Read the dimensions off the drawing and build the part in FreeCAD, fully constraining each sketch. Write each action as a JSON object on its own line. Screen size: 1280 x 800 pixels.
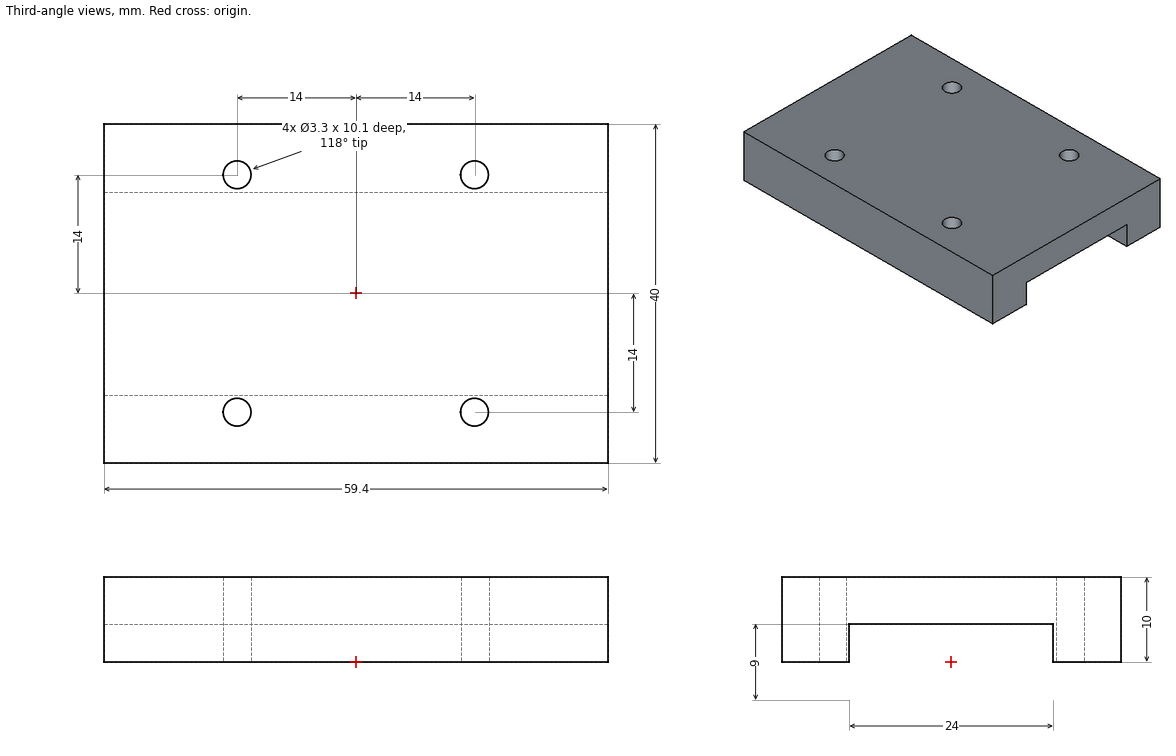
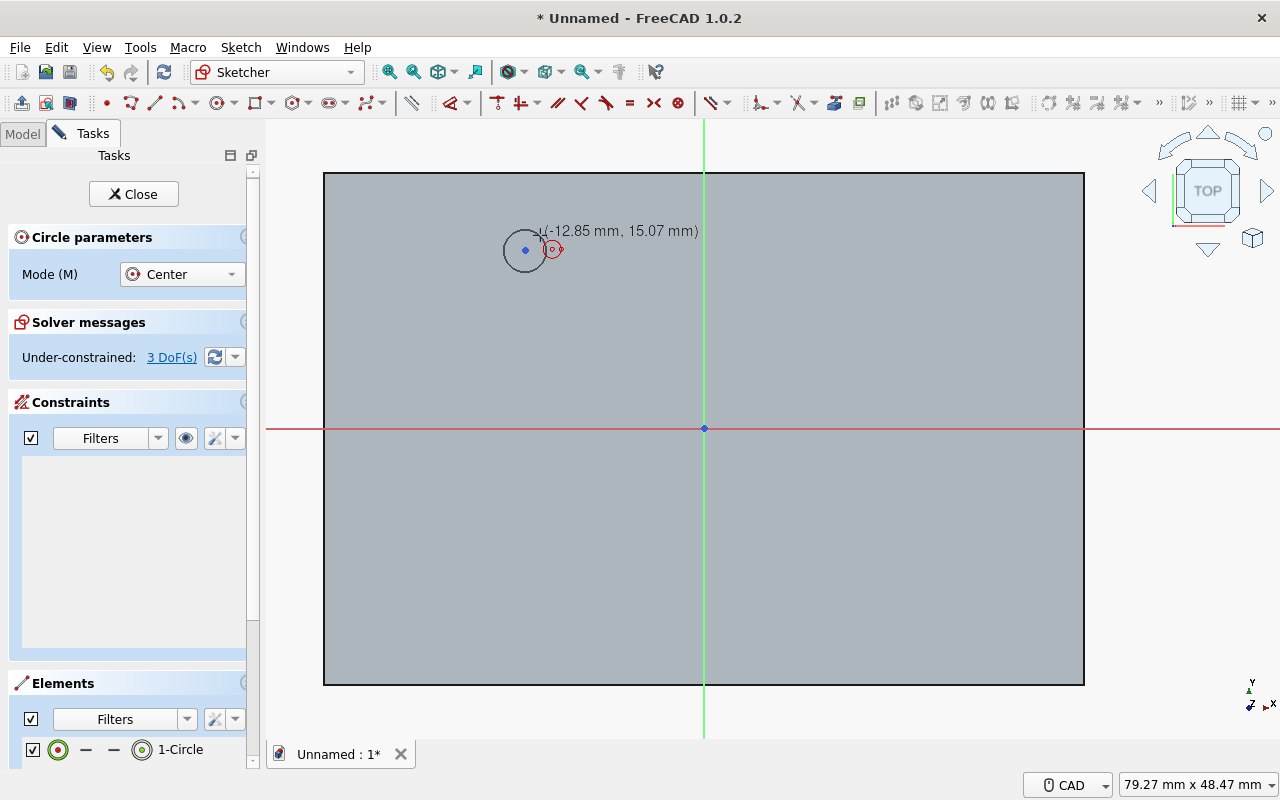
{"action": "left_click", "coordinate": [883, 250]}
{"action": "left_click", "coordinate": [898, 235]}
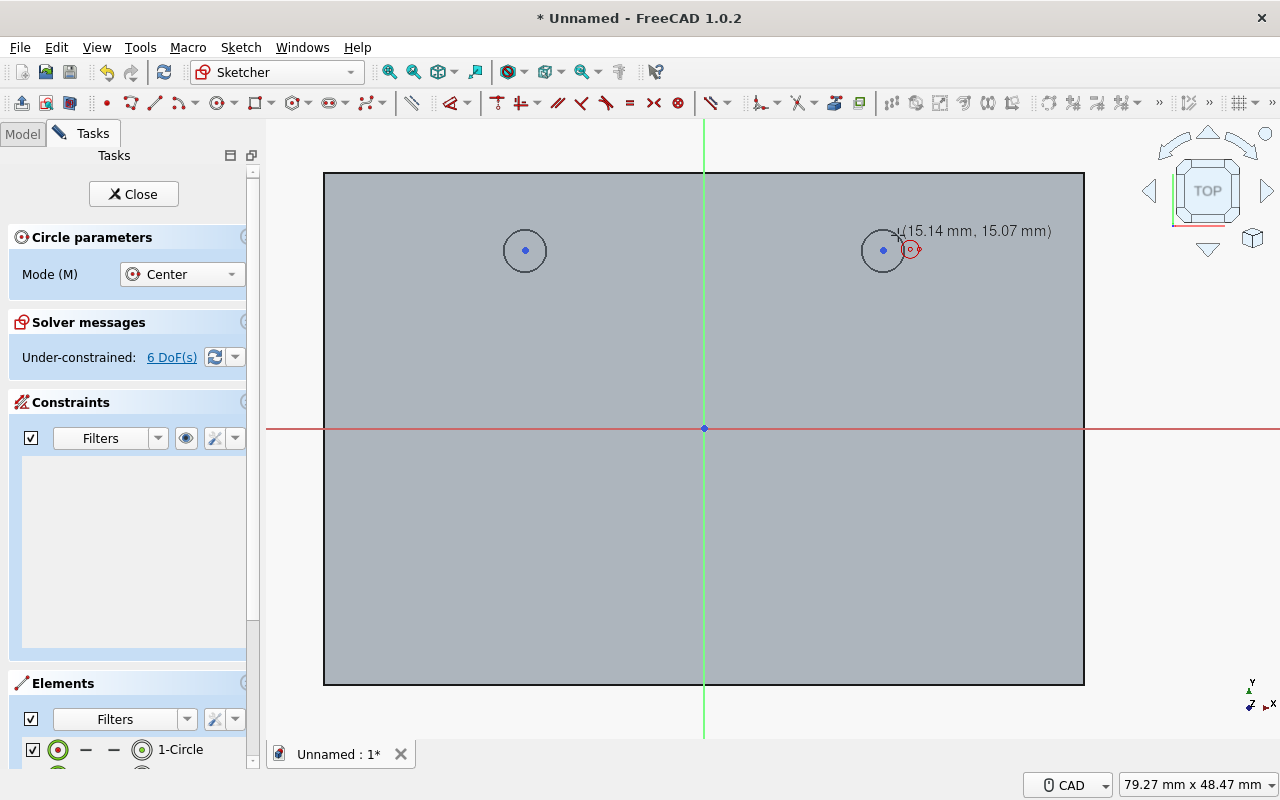
{"action": "left_click", "coordinate": [883, 608]}
{"action": "left_click", "coordinate": [898, 593]}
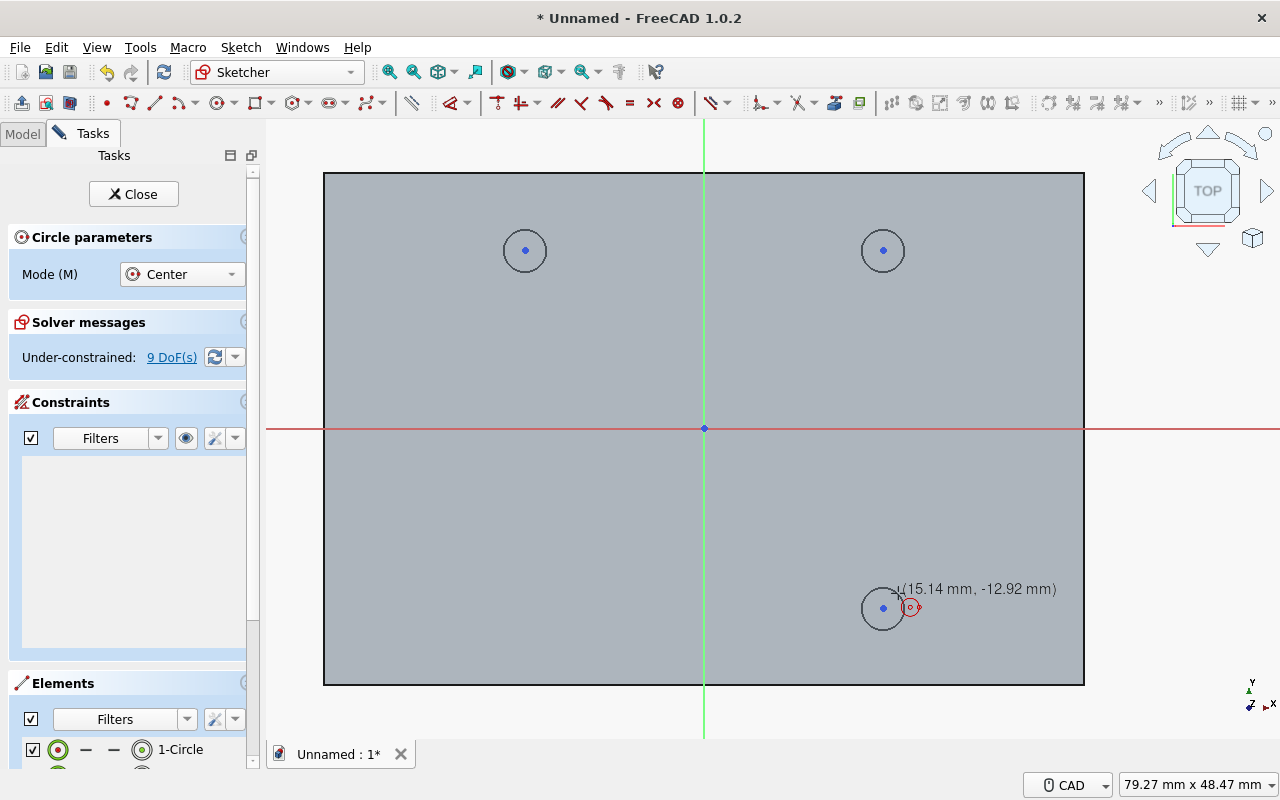
{"action": "left_click", "coordinate": [525, 608]}
{"action": "left_click", "coordinate": [540, 593]}
{"action": "key", "text": "Escape"}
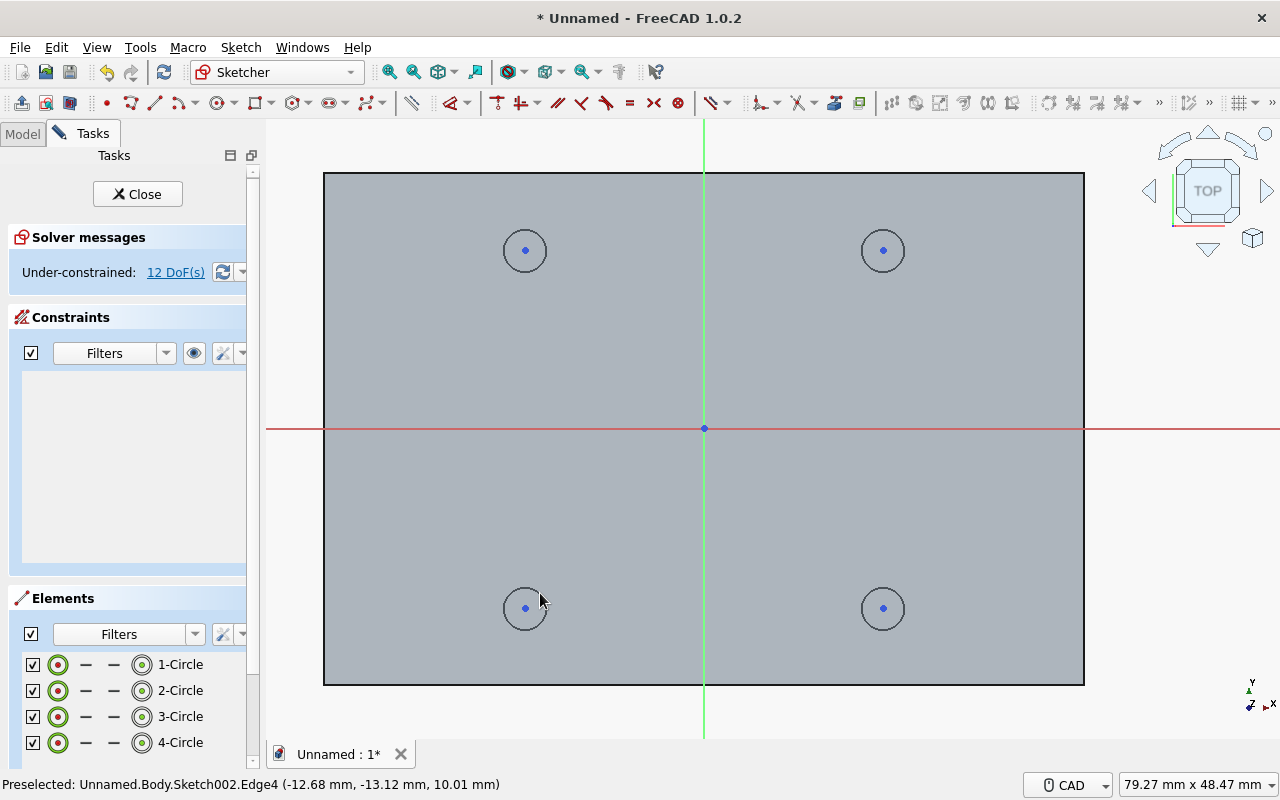
{"action": "left_click", "coordinate": [540, 236]}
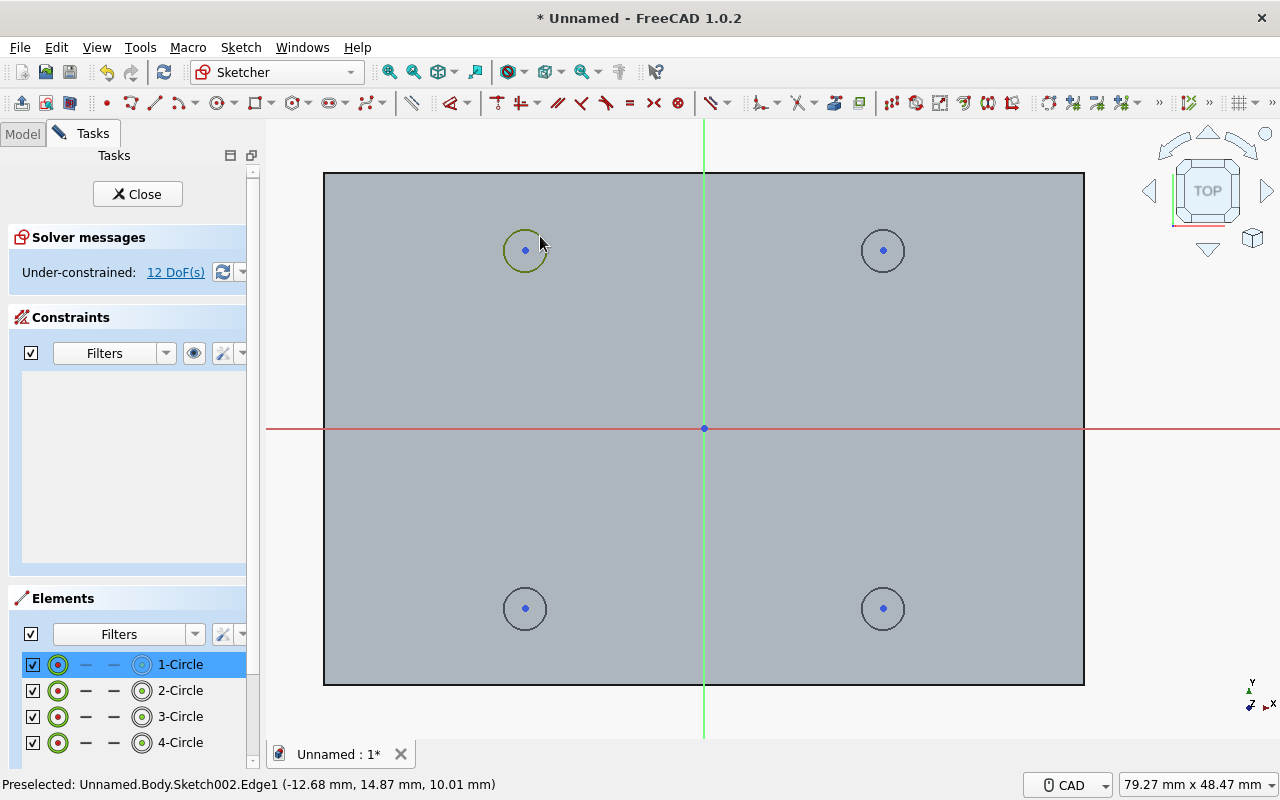
{"action": "left_click", "coordinate": [898, 236]}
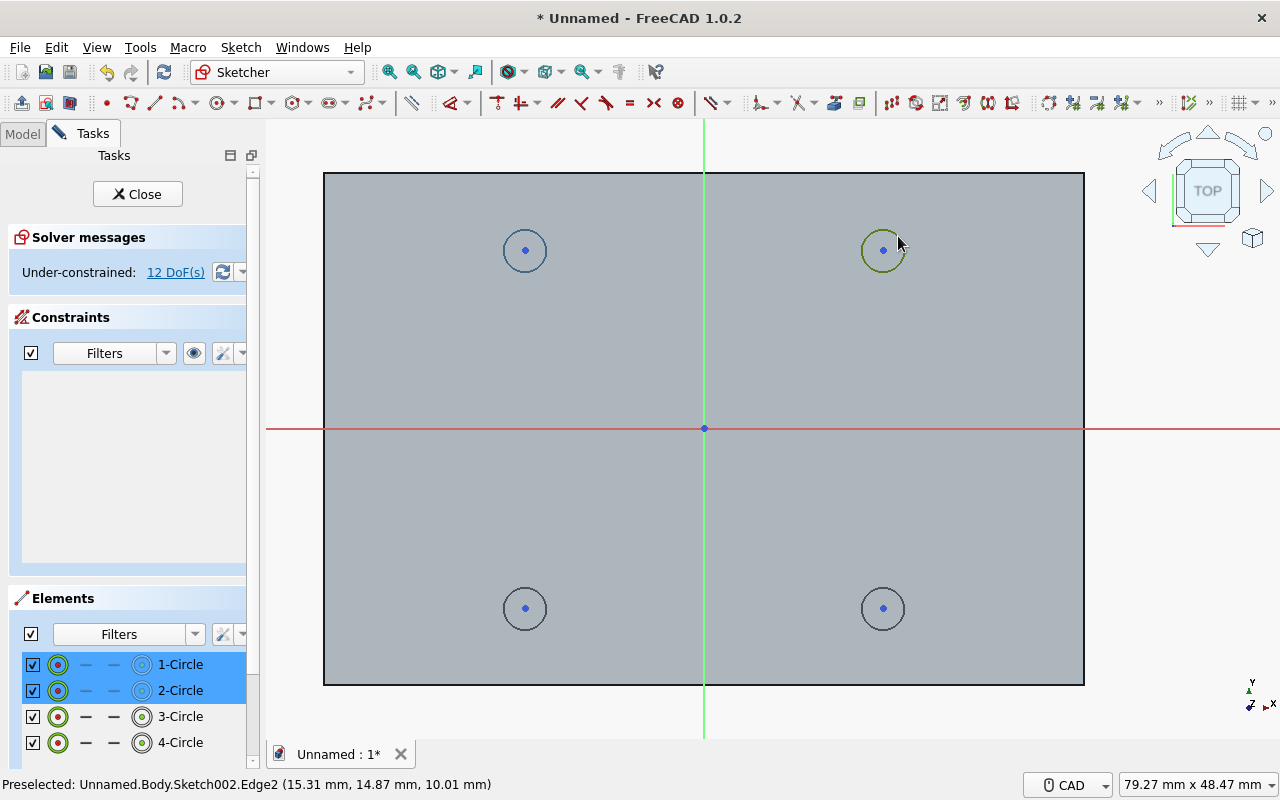
{"action": "left_click", "coordinate": [898, 594]}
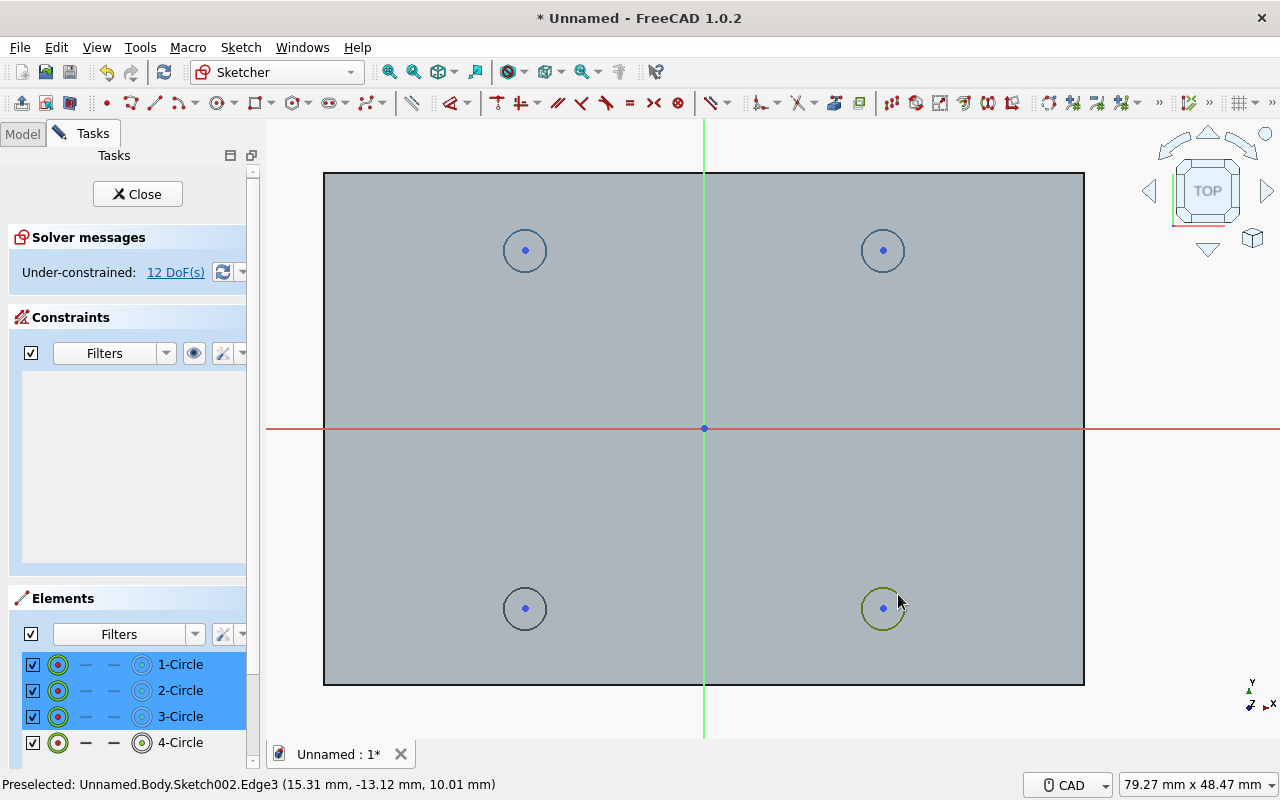
{"action": "left_click", "coordinate": [540, 594]}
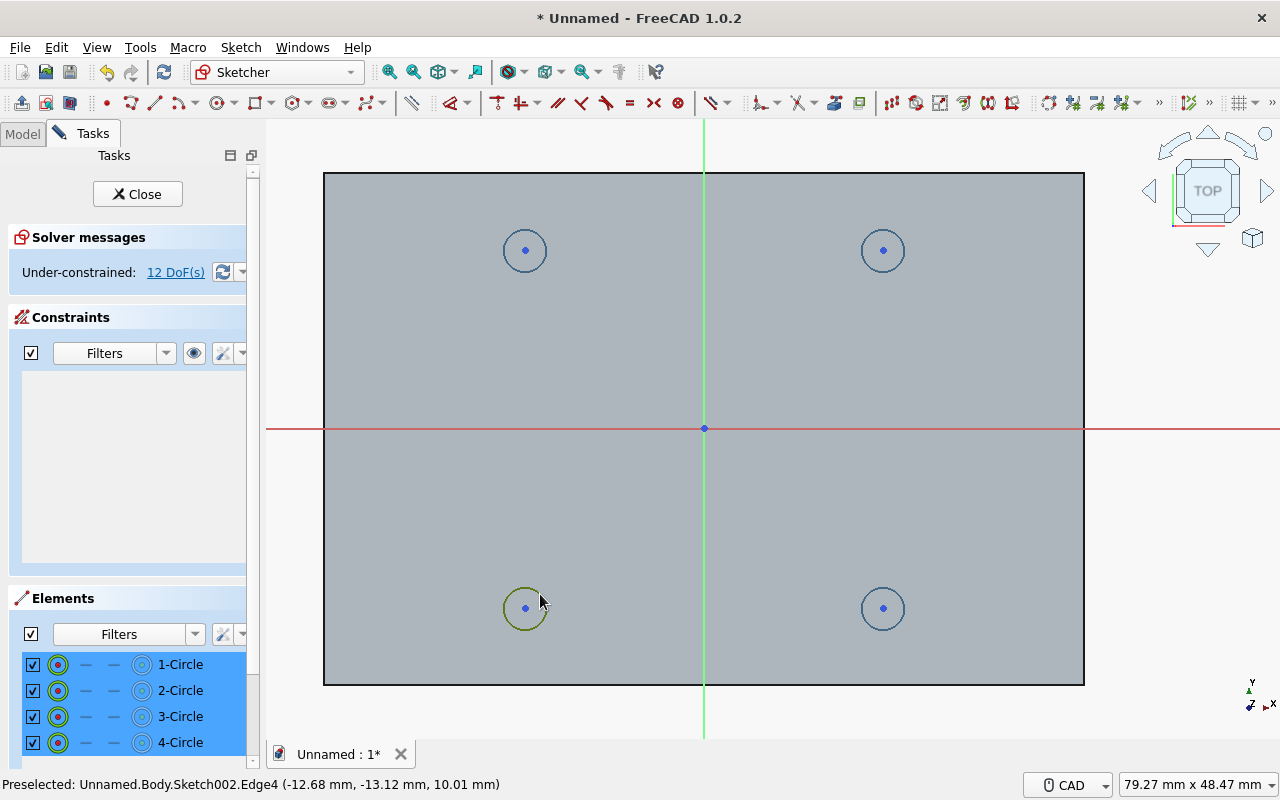
{"action": "key", "text": "e"}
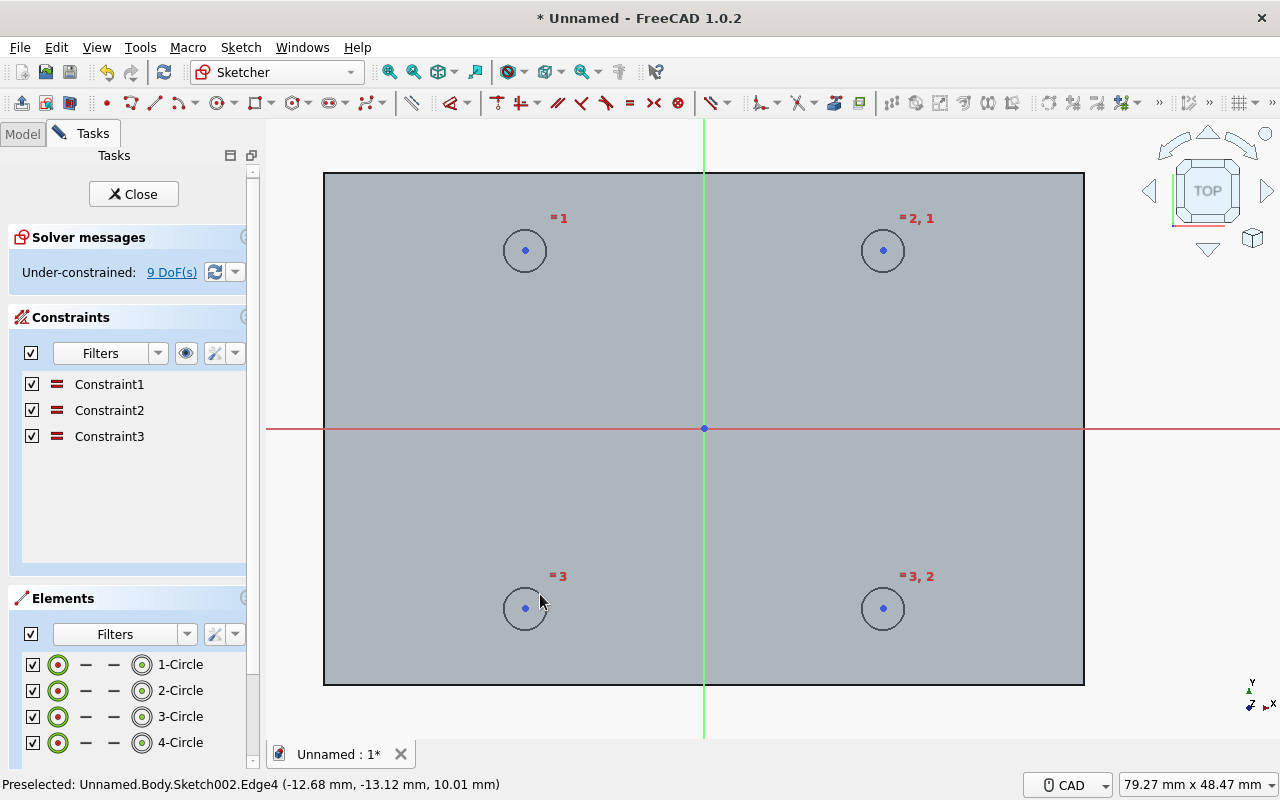
{"action": "left_click", "coordinate": [525, 251]}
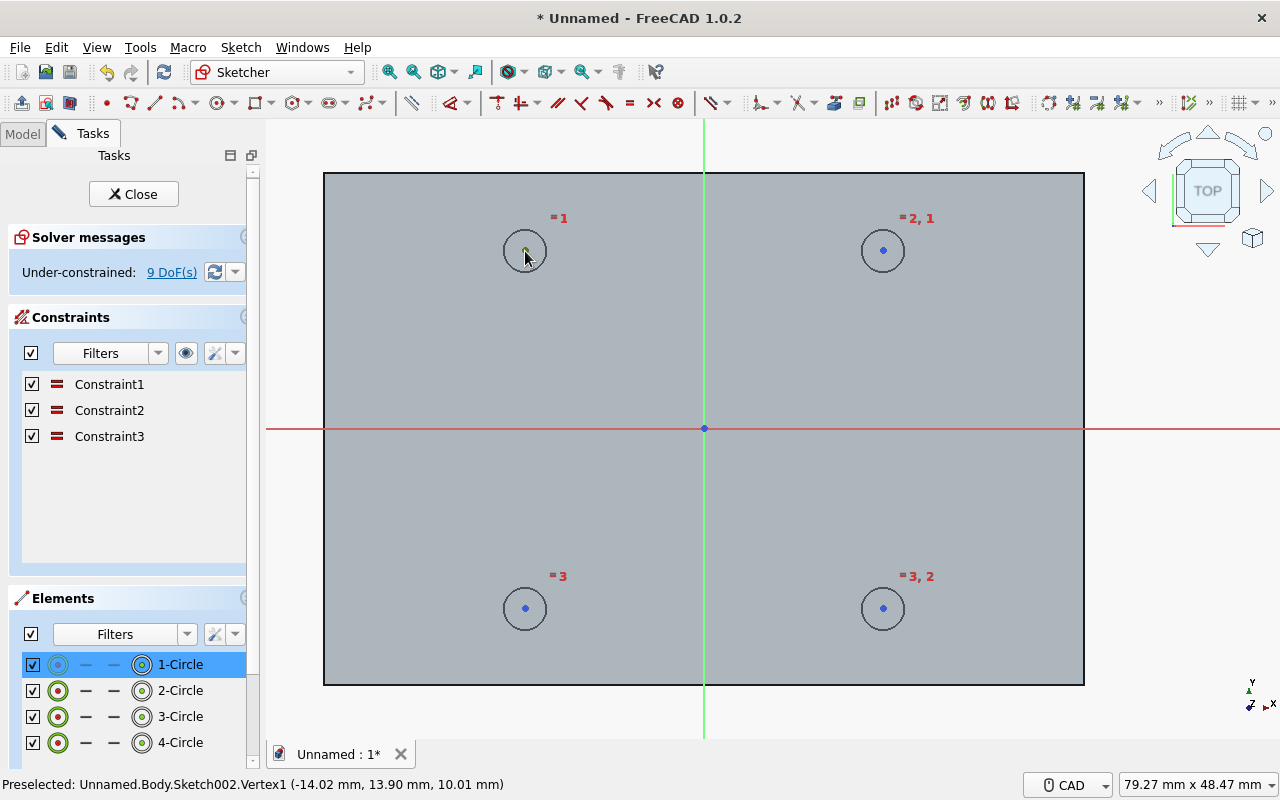
{"action": "left_click", "coordinate": [883, 251]}